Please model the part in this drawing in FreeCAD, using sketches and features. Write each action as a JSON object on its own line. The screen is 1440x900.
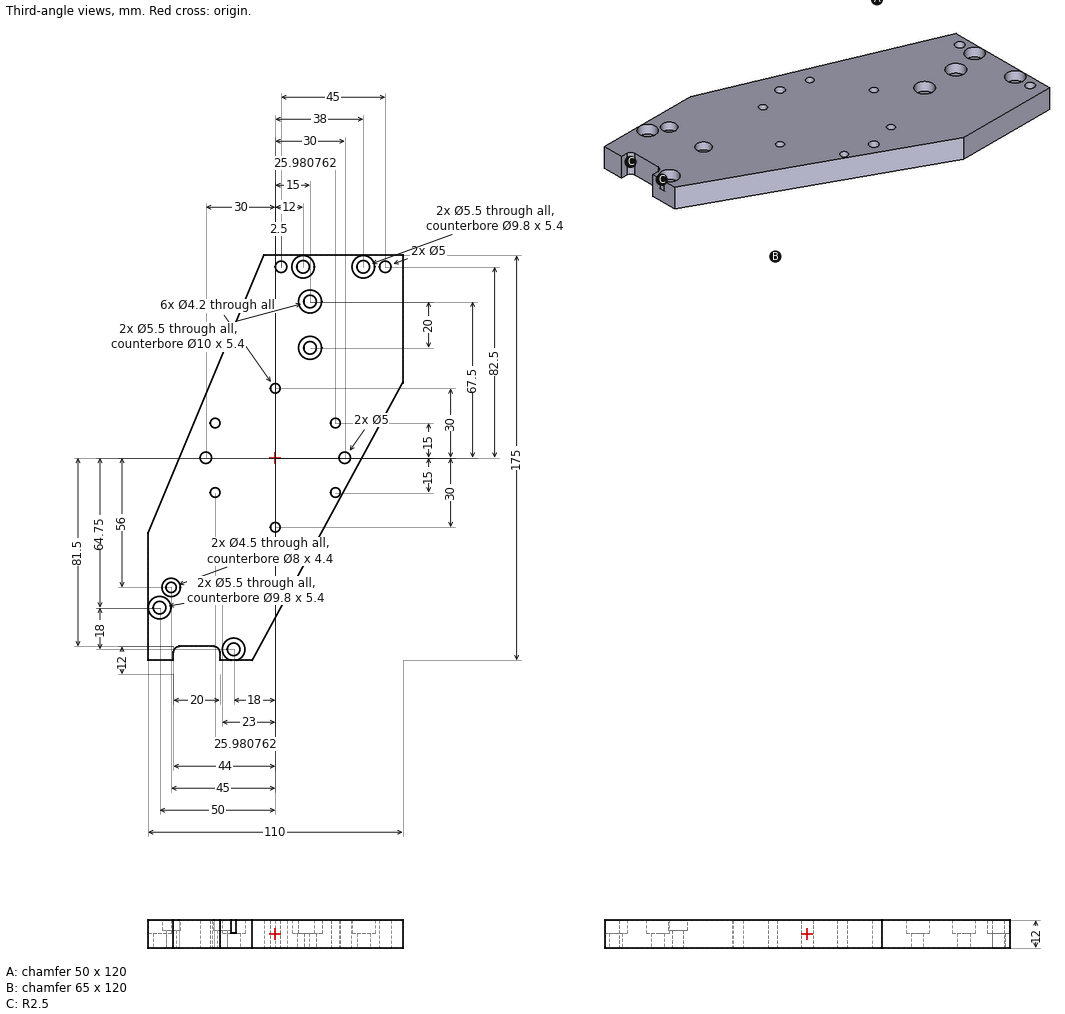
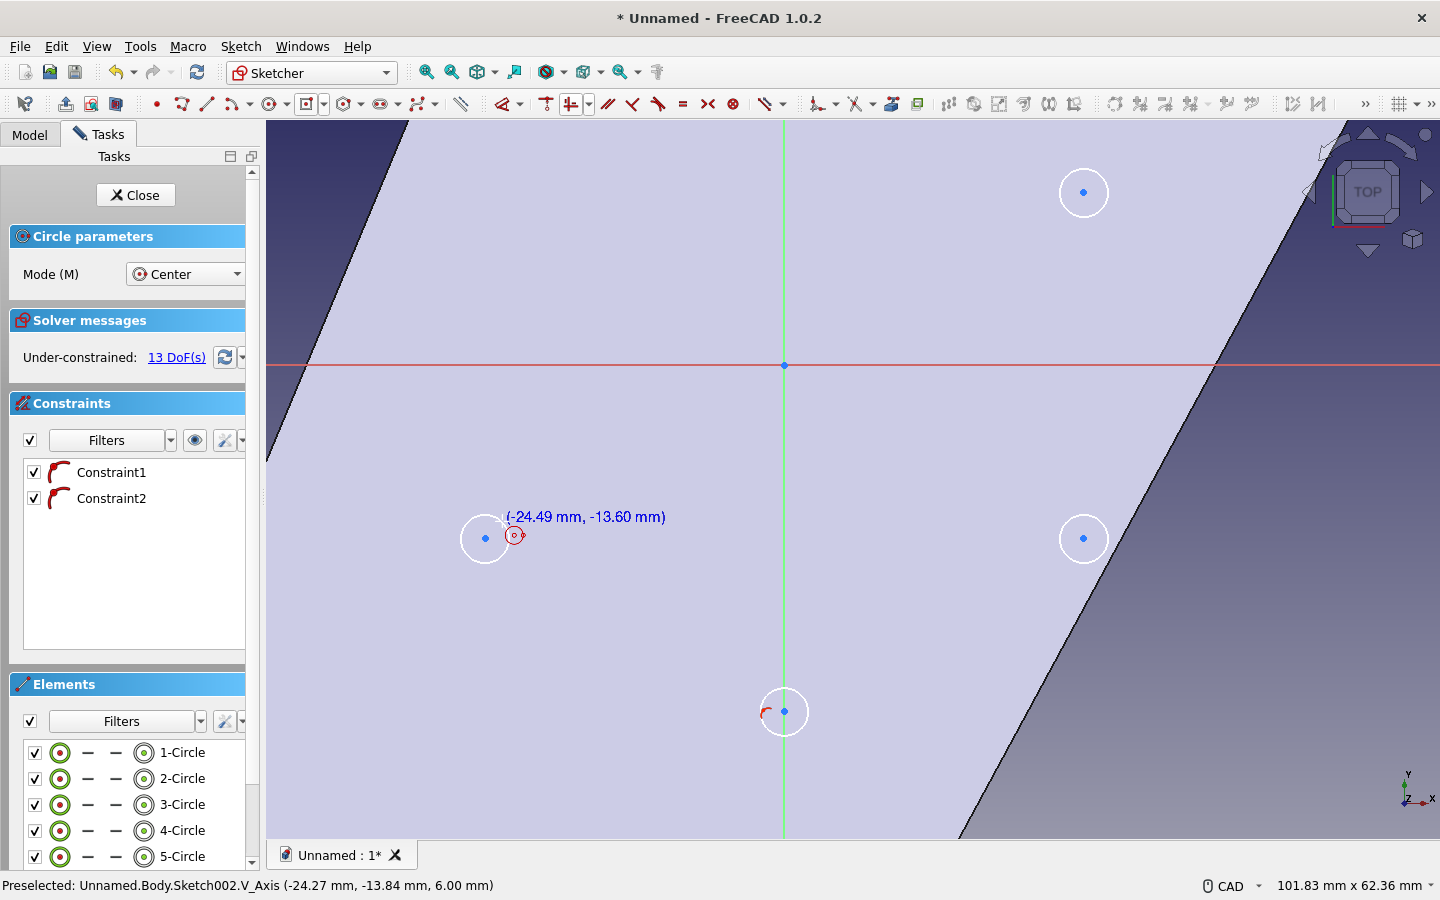
{"action": "left_click", "coordinate": [485, 192]}
{"action": "left_click", "coordinate": [502, 175]}
{"action": "key", "text": "Escape"}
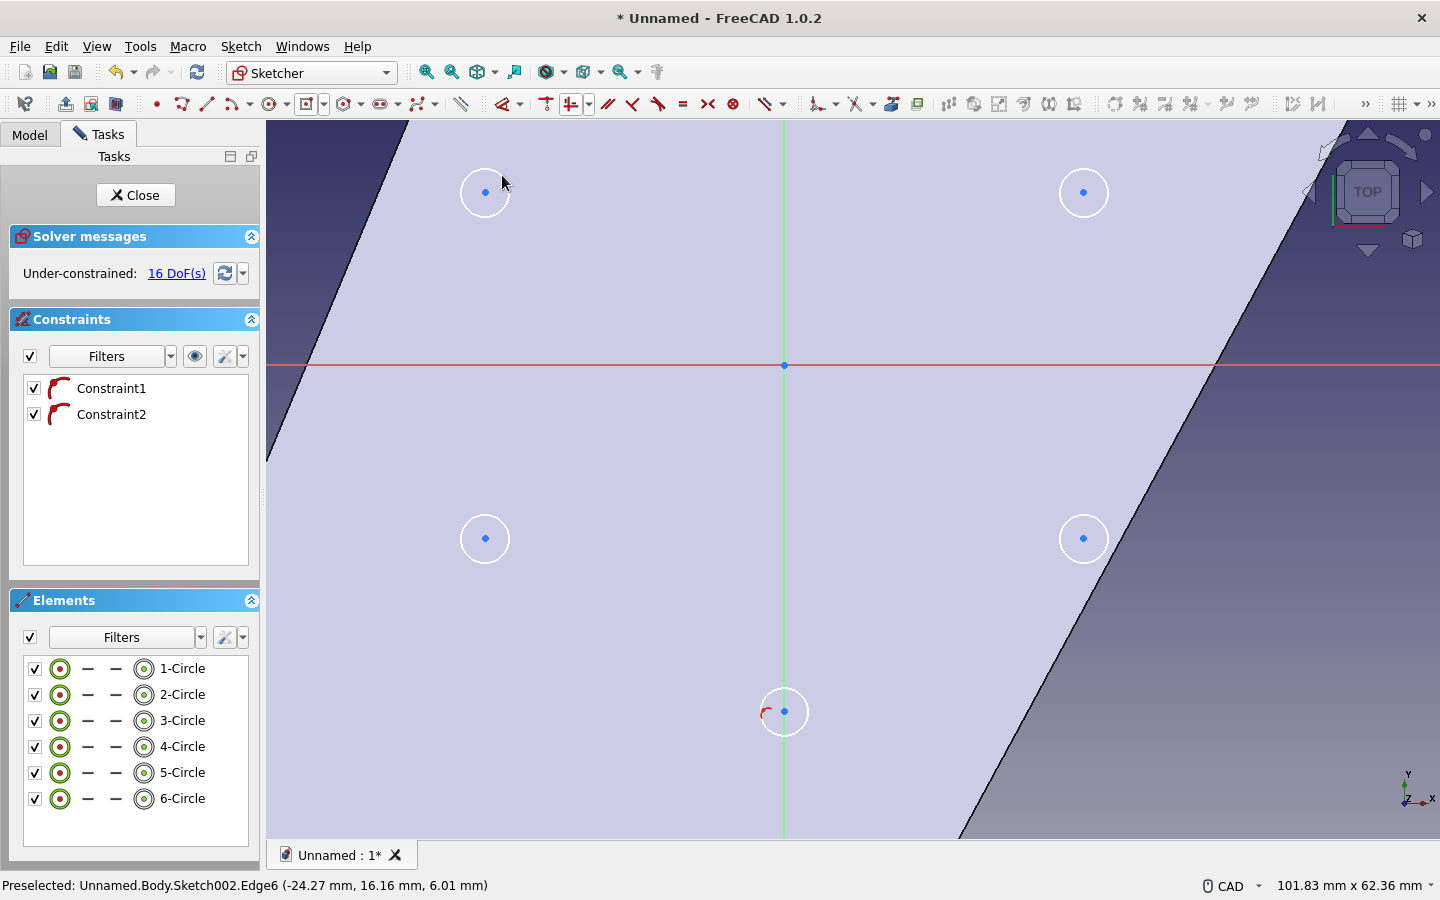
{"action": "scroll", "coordinate": [785, 712], "scroll_direction": "down", "scroll_amount": 2}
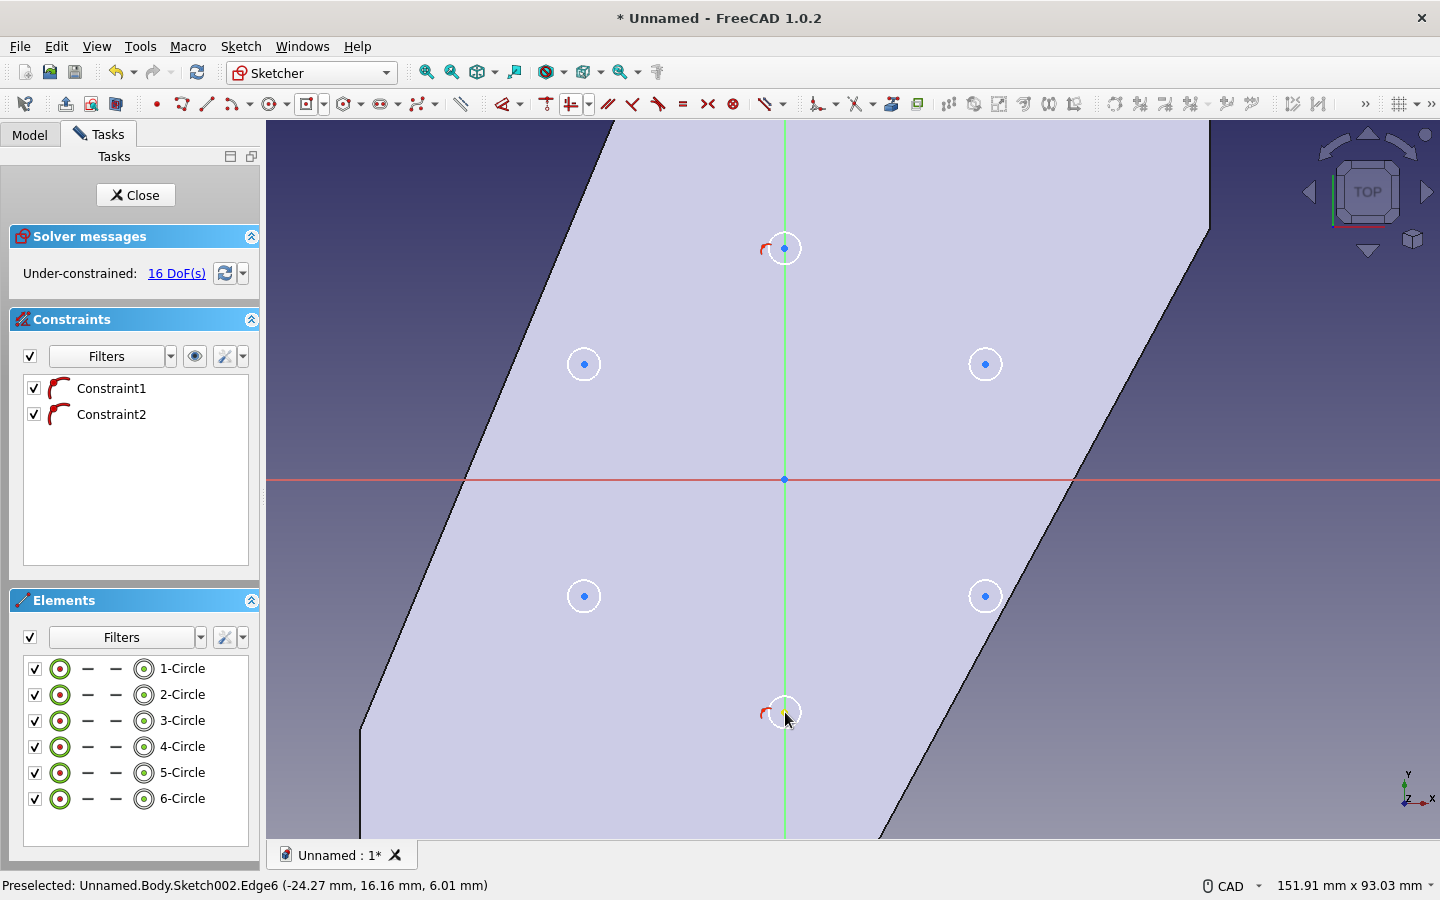
{"action": "scroll", "coordinate": [796, 237], "scroll_direction": "up", "scroll_amount": 2}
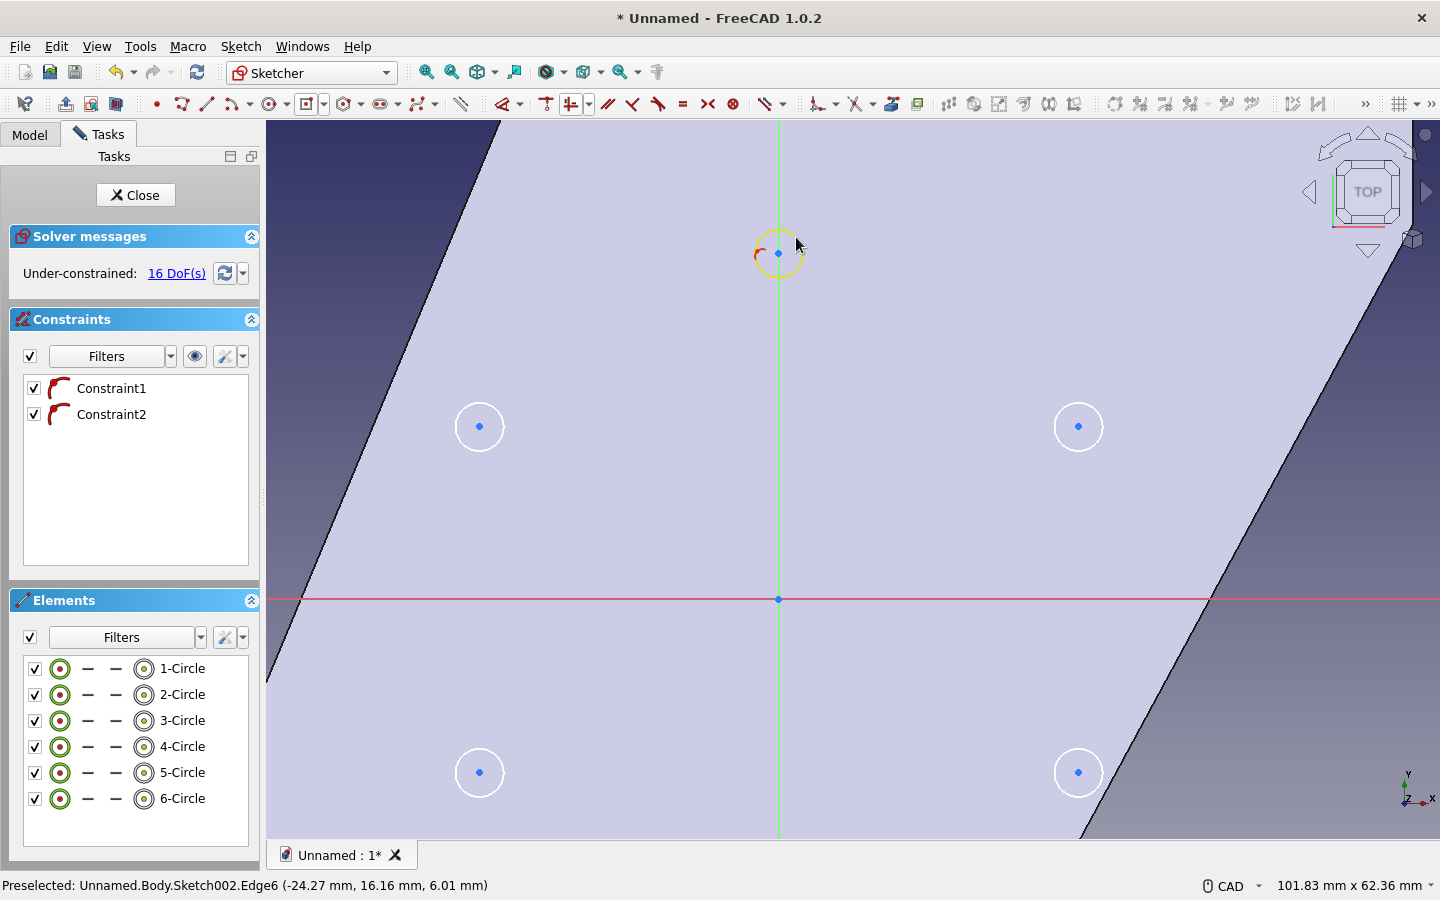
{"action": "left_click", "coordinate": [796, 237]}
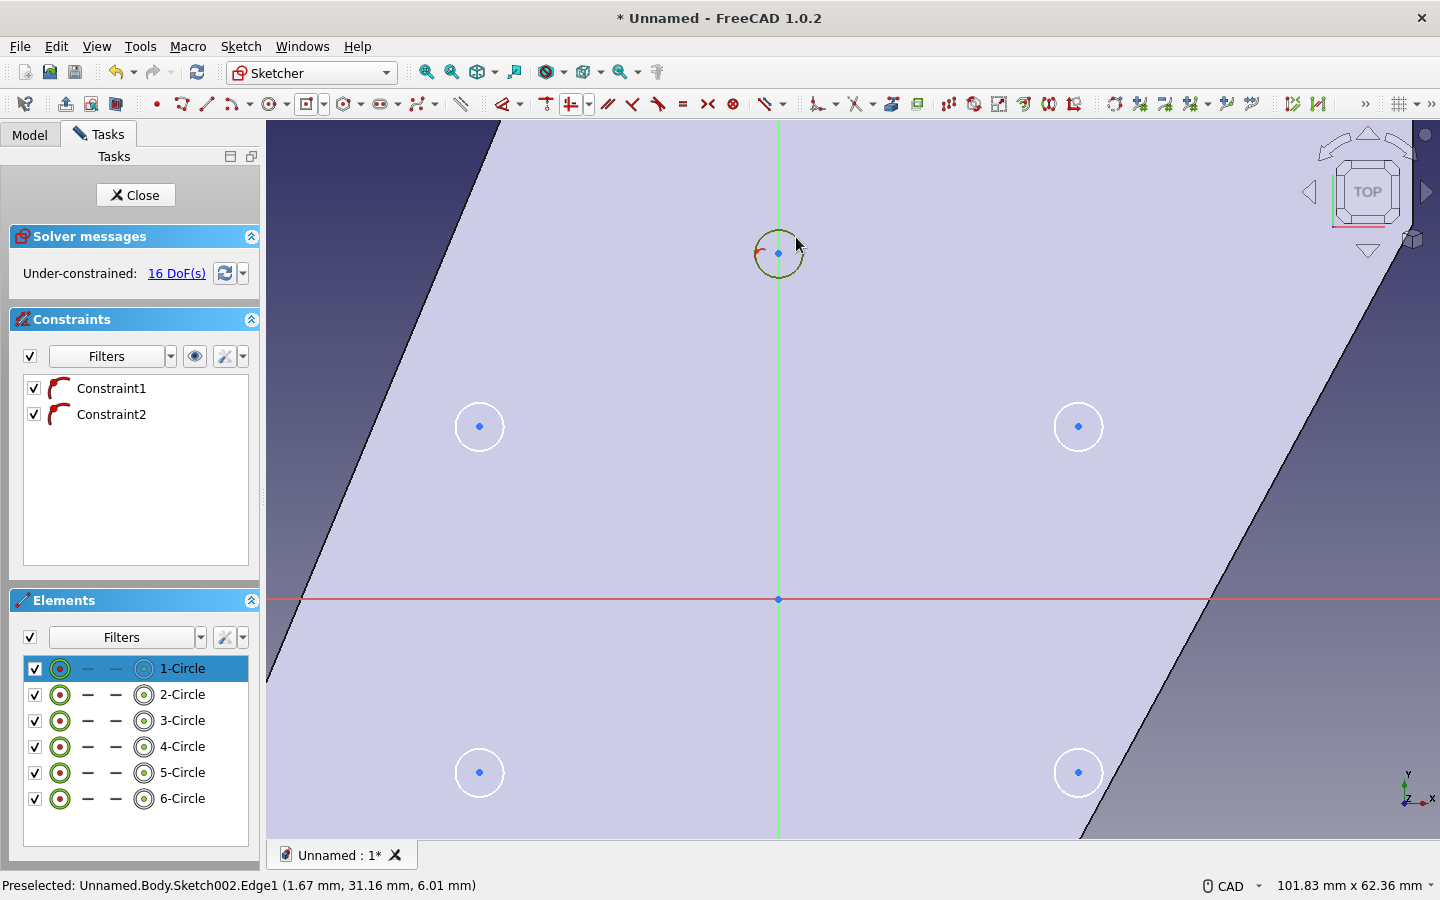
{"action": "left_click", "coordinate": [1096, 410]}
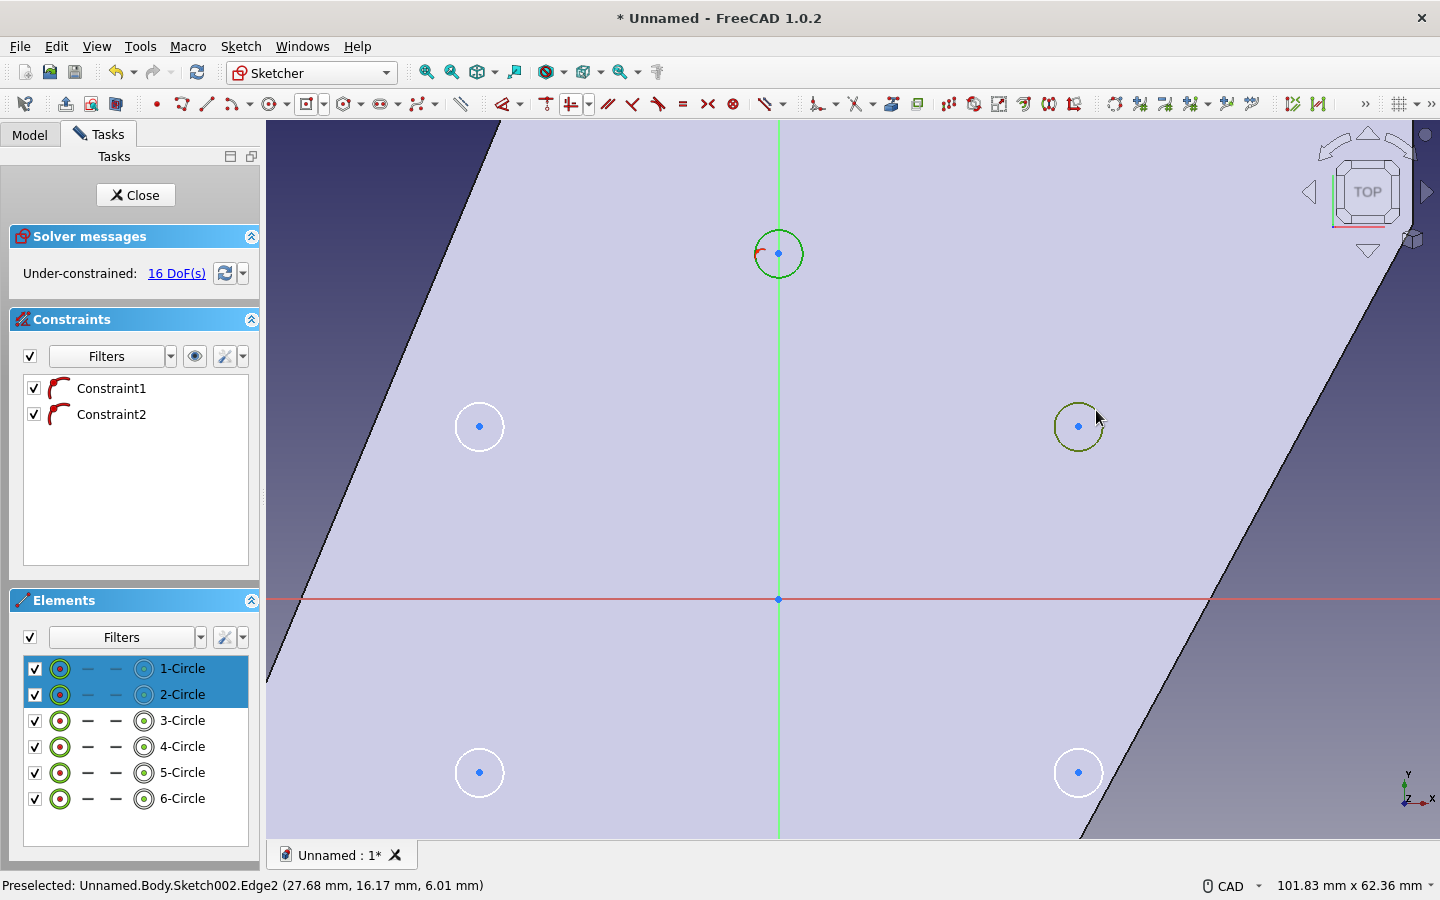
{"action": "left_click", "coordinate": [1096, 756]}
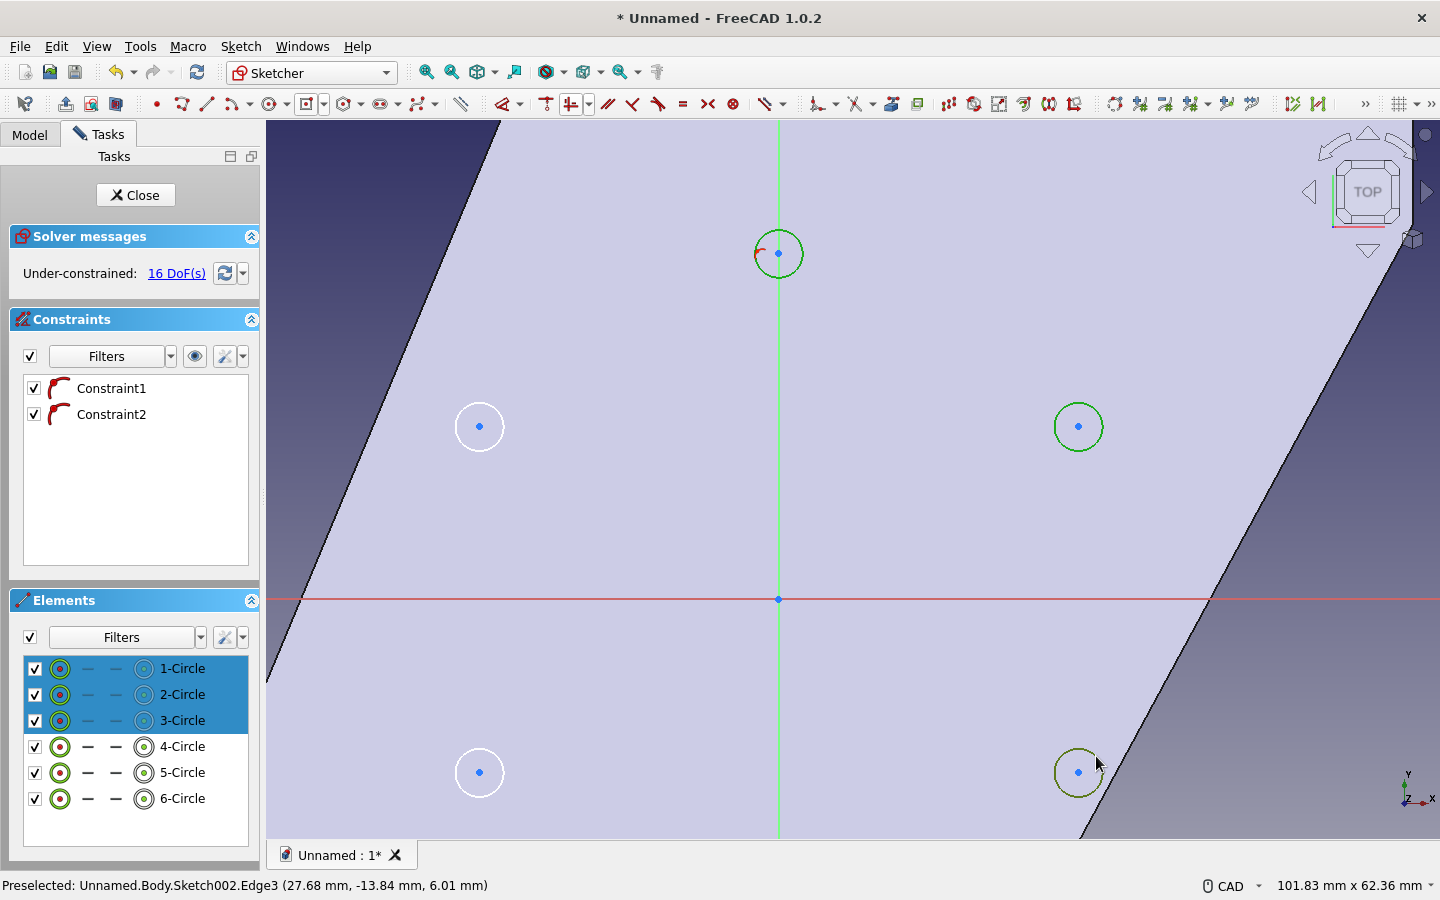
{"action": "scroll", "coordinate": [796, 236], "scroll_direction": "down", "scroll_amount": 2}